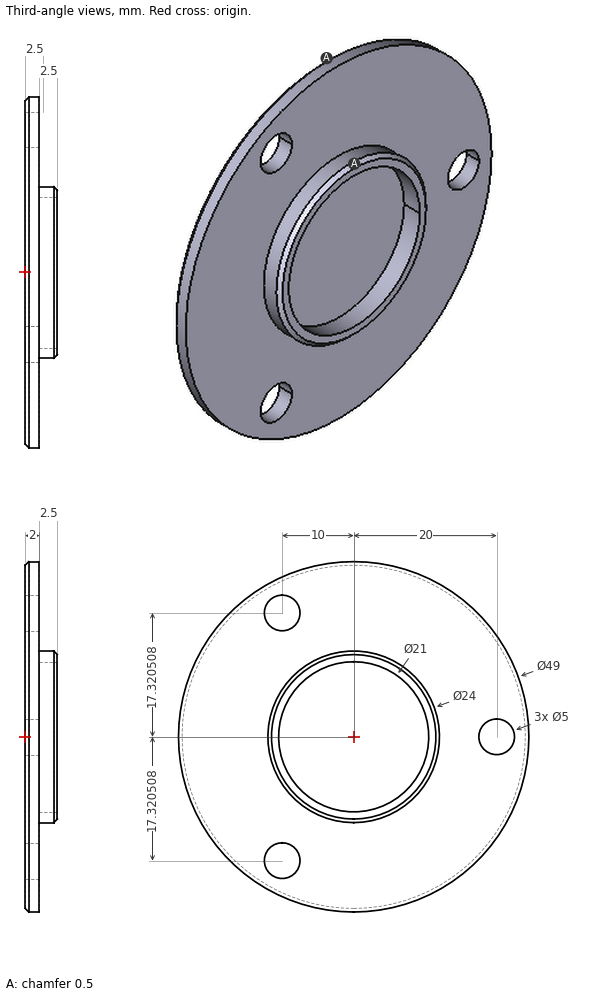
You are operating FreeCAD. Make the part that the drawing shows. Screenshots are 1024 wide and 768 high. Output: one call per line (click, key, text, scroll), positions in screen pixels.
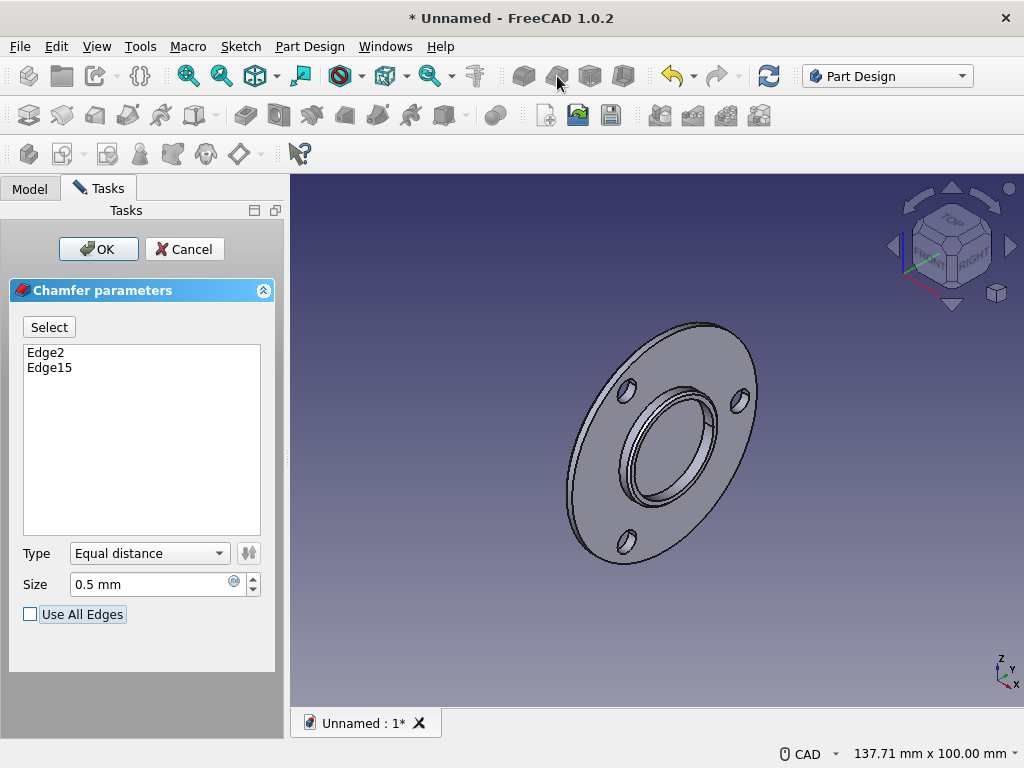
click(99, 249)